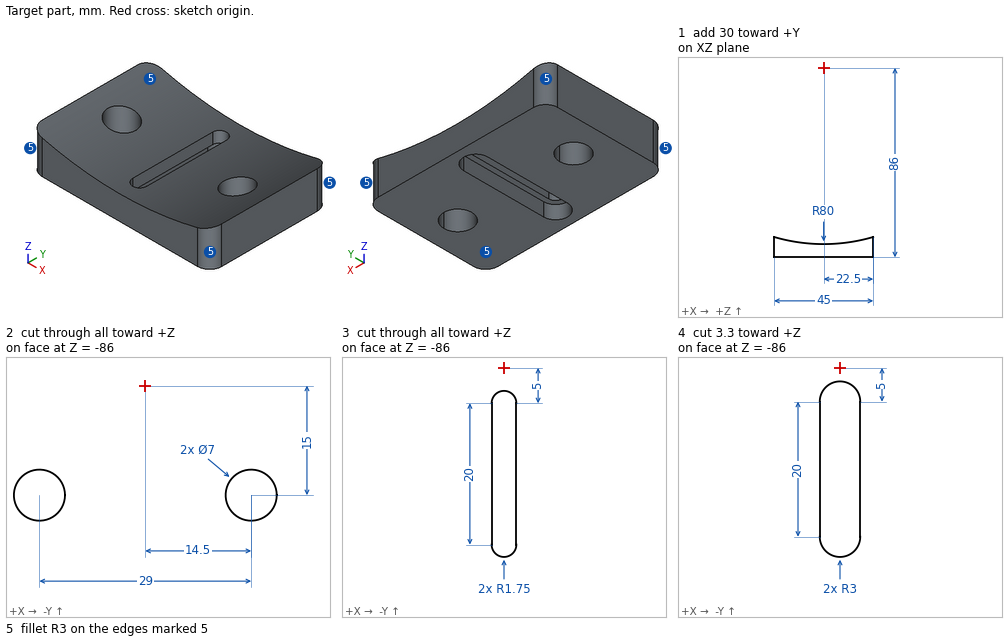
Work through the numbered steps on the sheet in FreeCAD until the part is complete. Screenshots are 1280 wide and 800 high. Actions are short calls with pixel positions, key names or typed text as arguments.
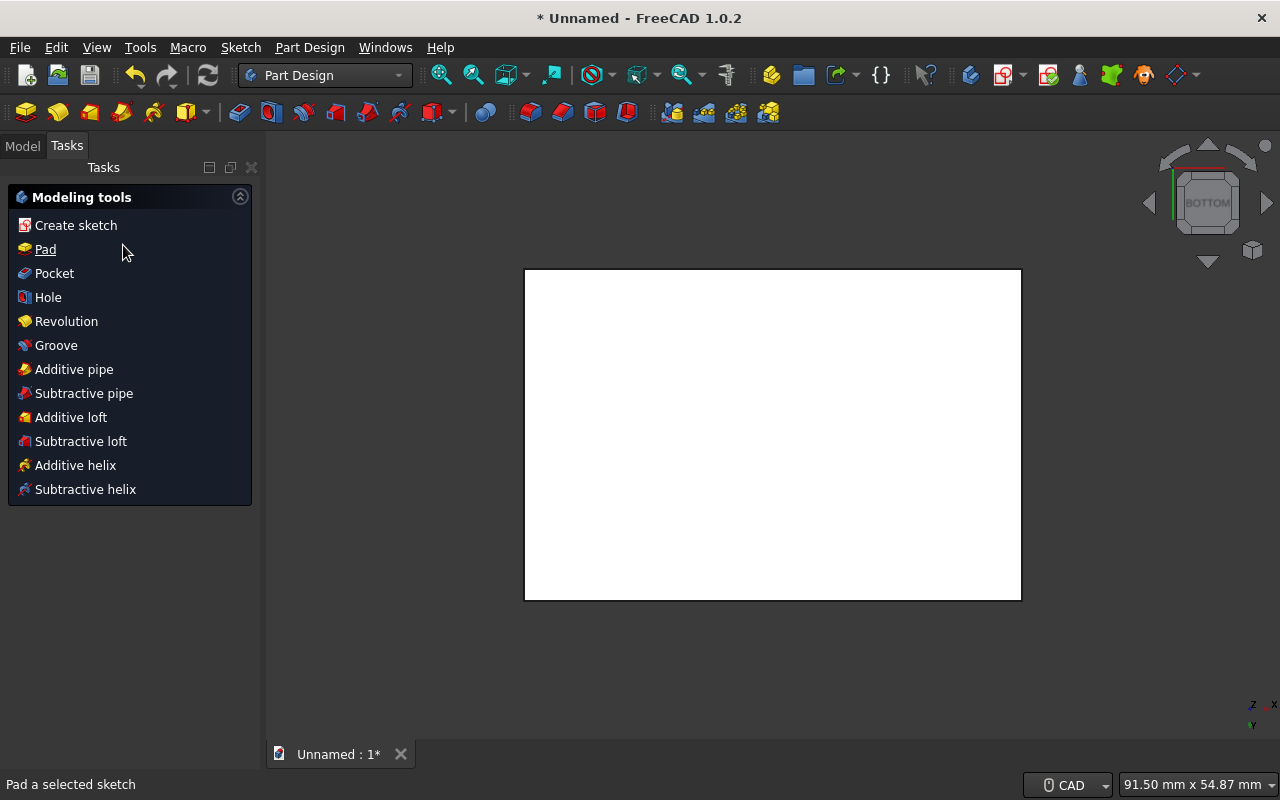
click(240, 112)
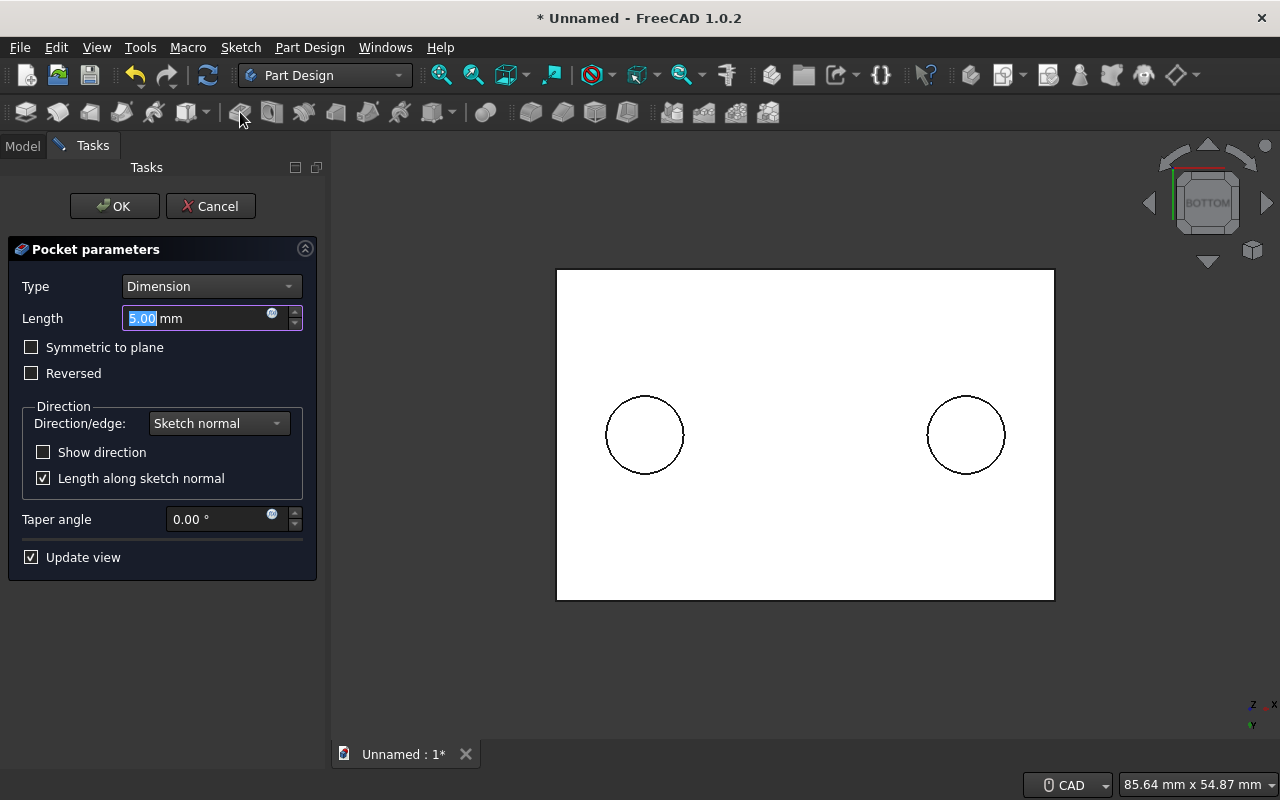
click(212, 286)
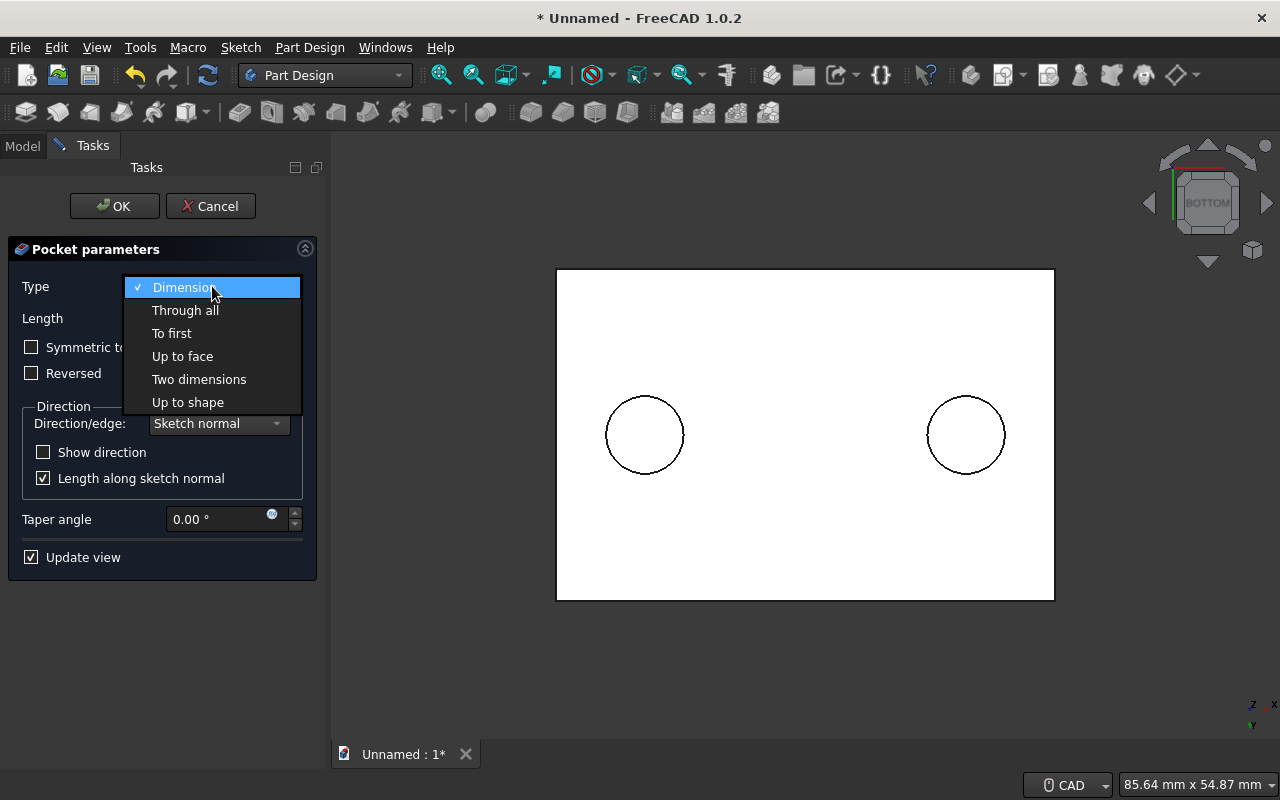
click(212, 310)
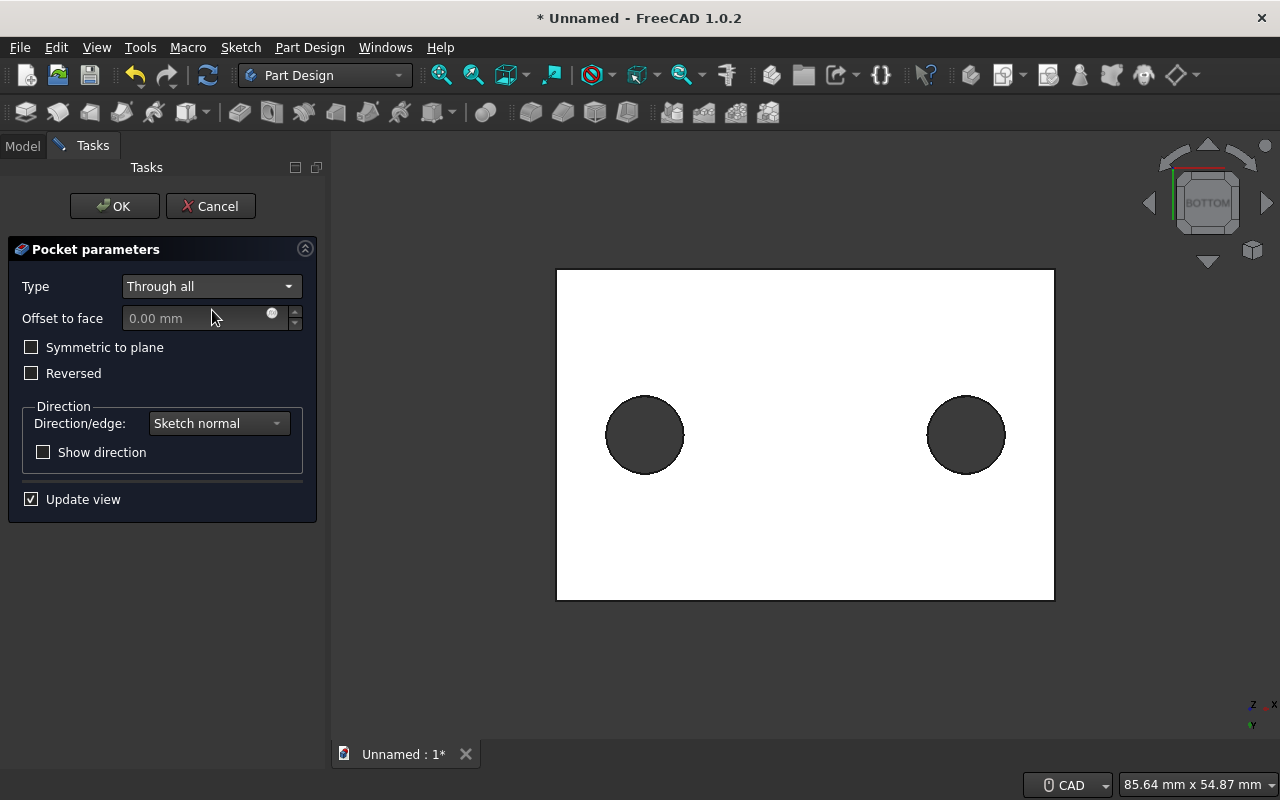
click(115, 206)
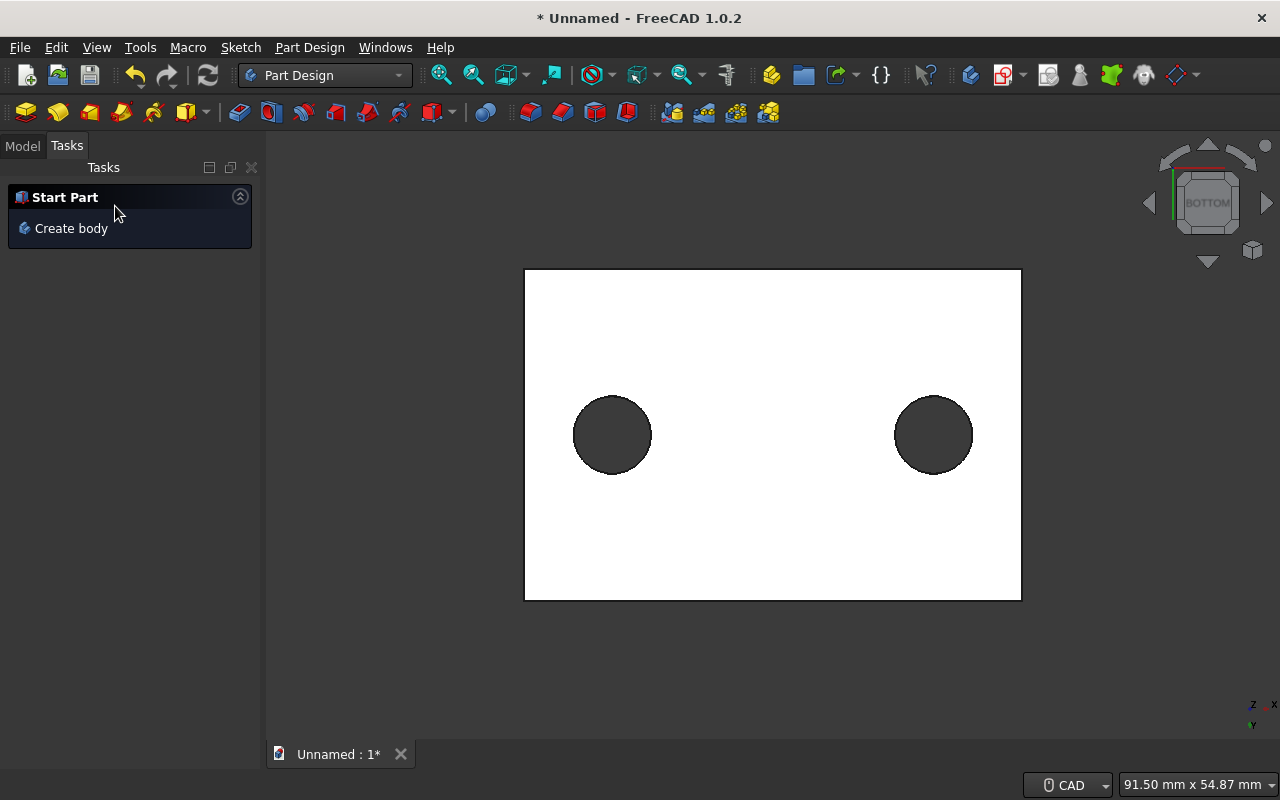
click(773, 434)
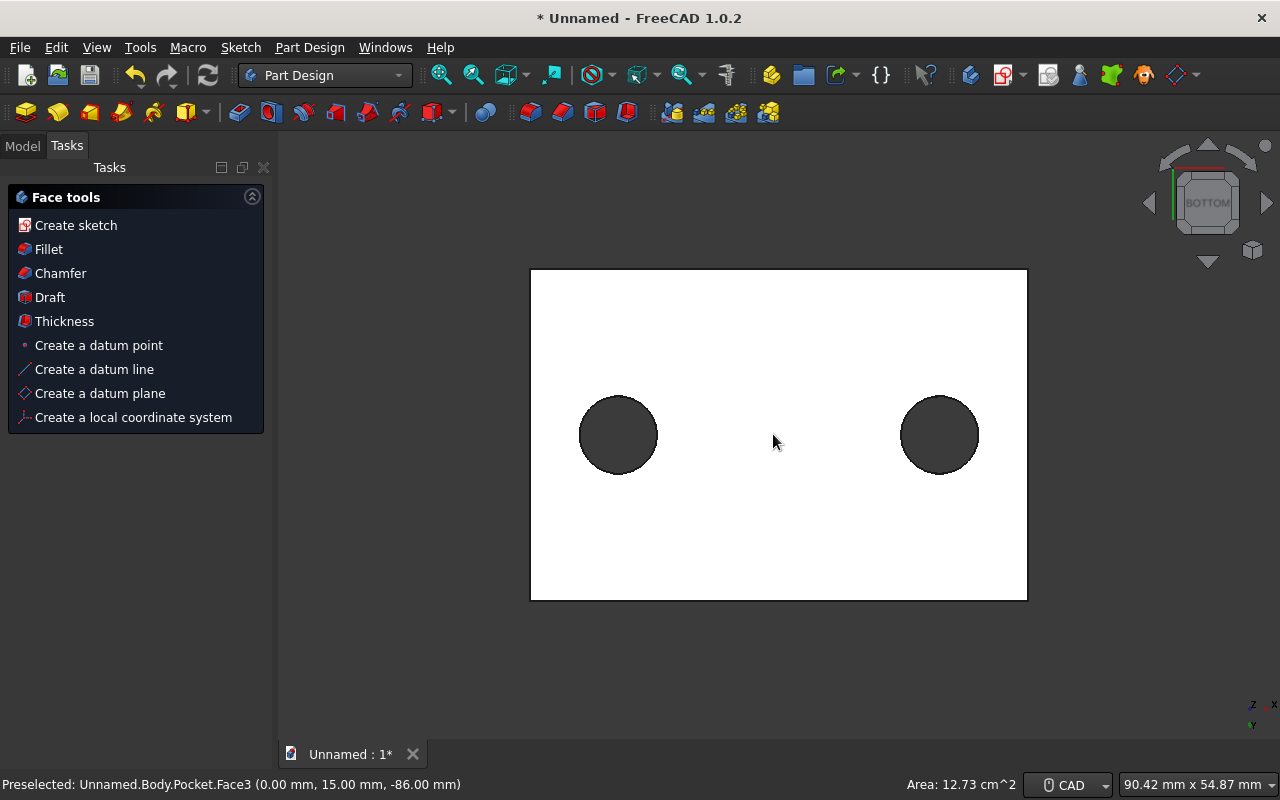
click(1004, 76)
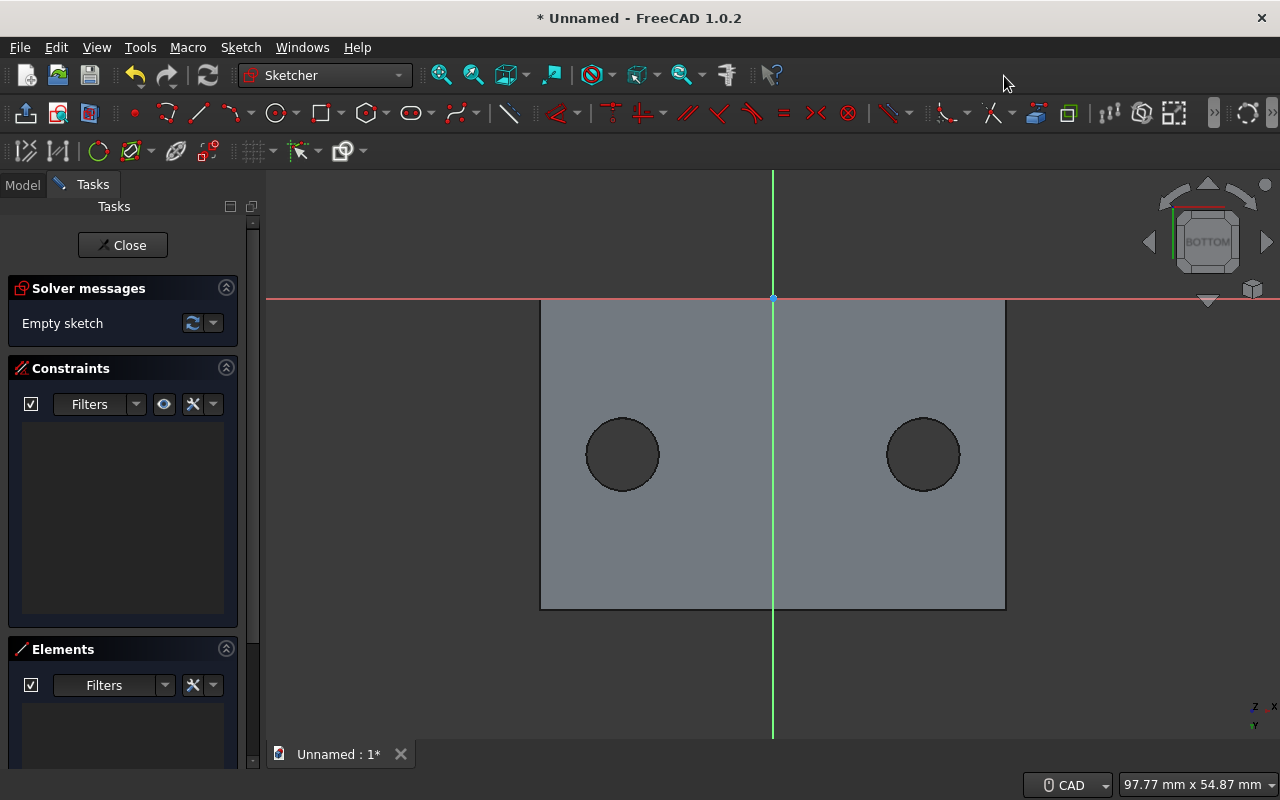
click(412, 114)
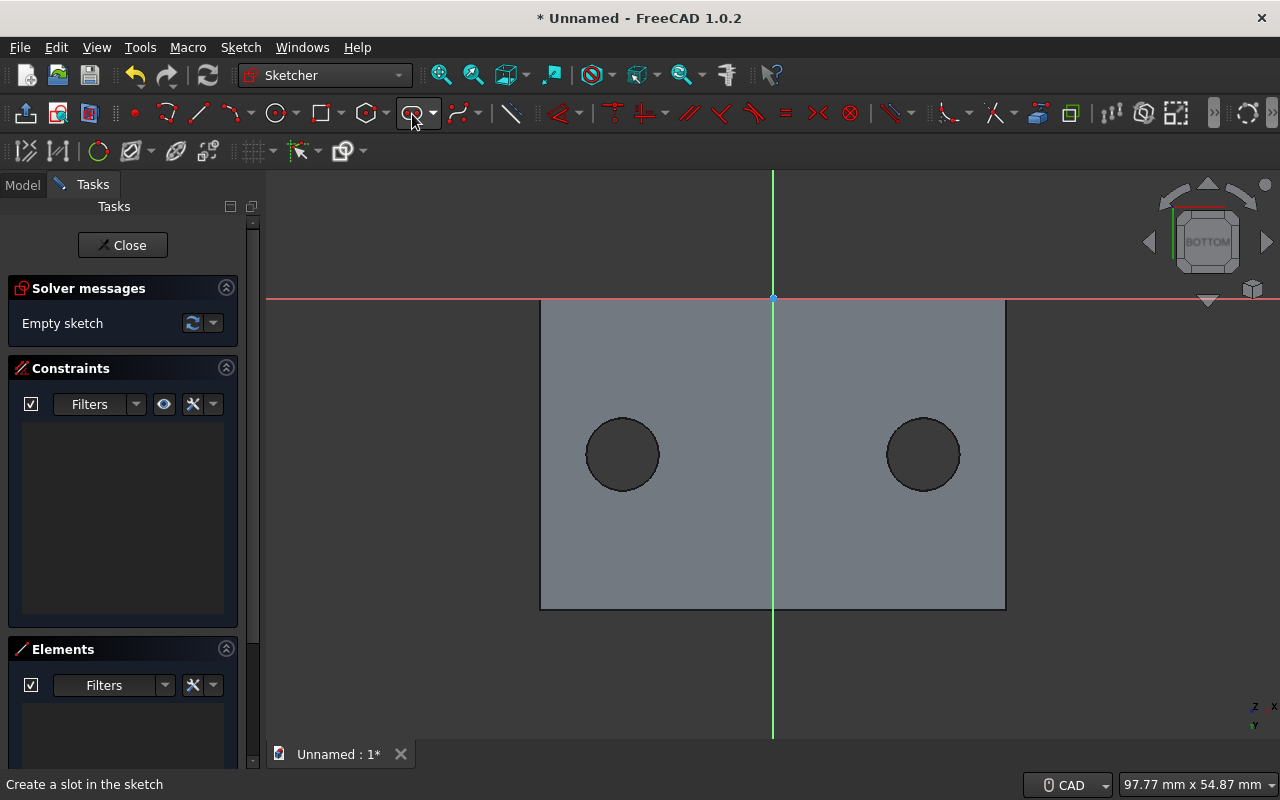
scroll(773, 558, up, 2)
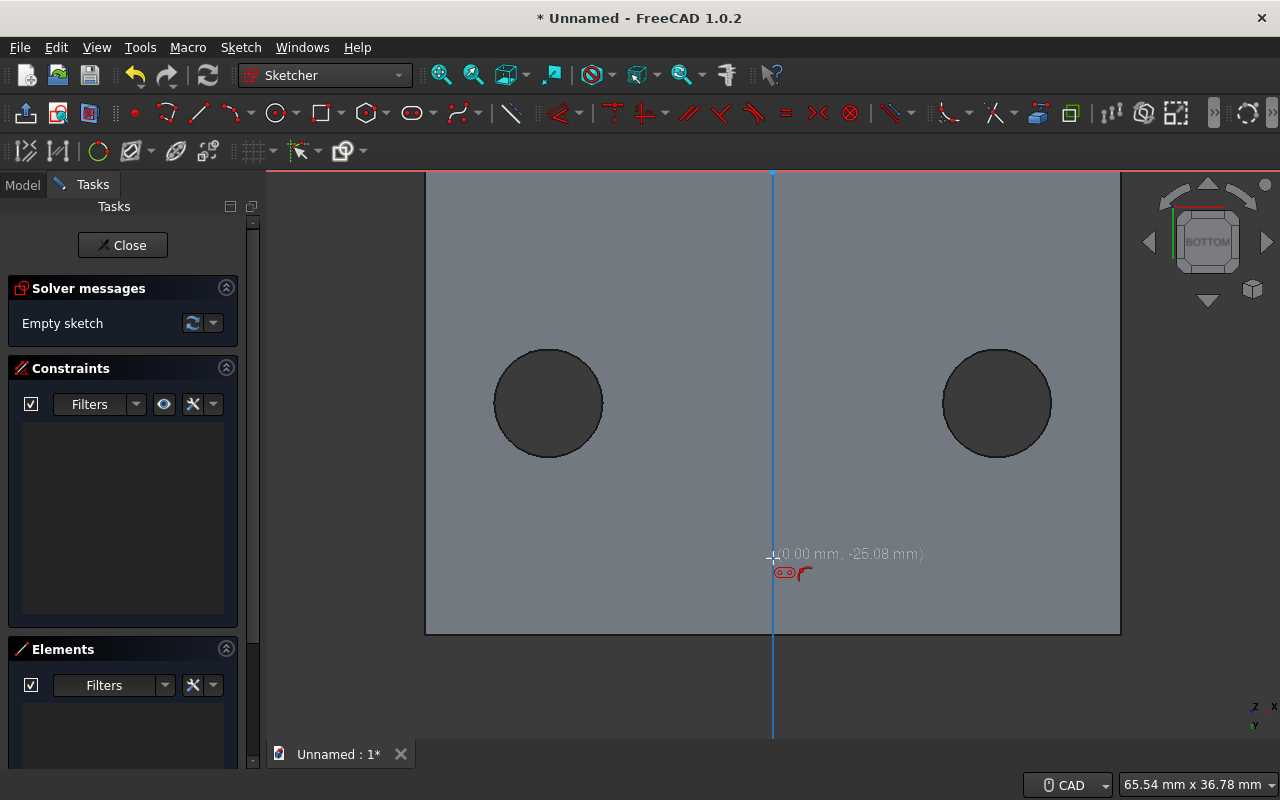
click(773, 558)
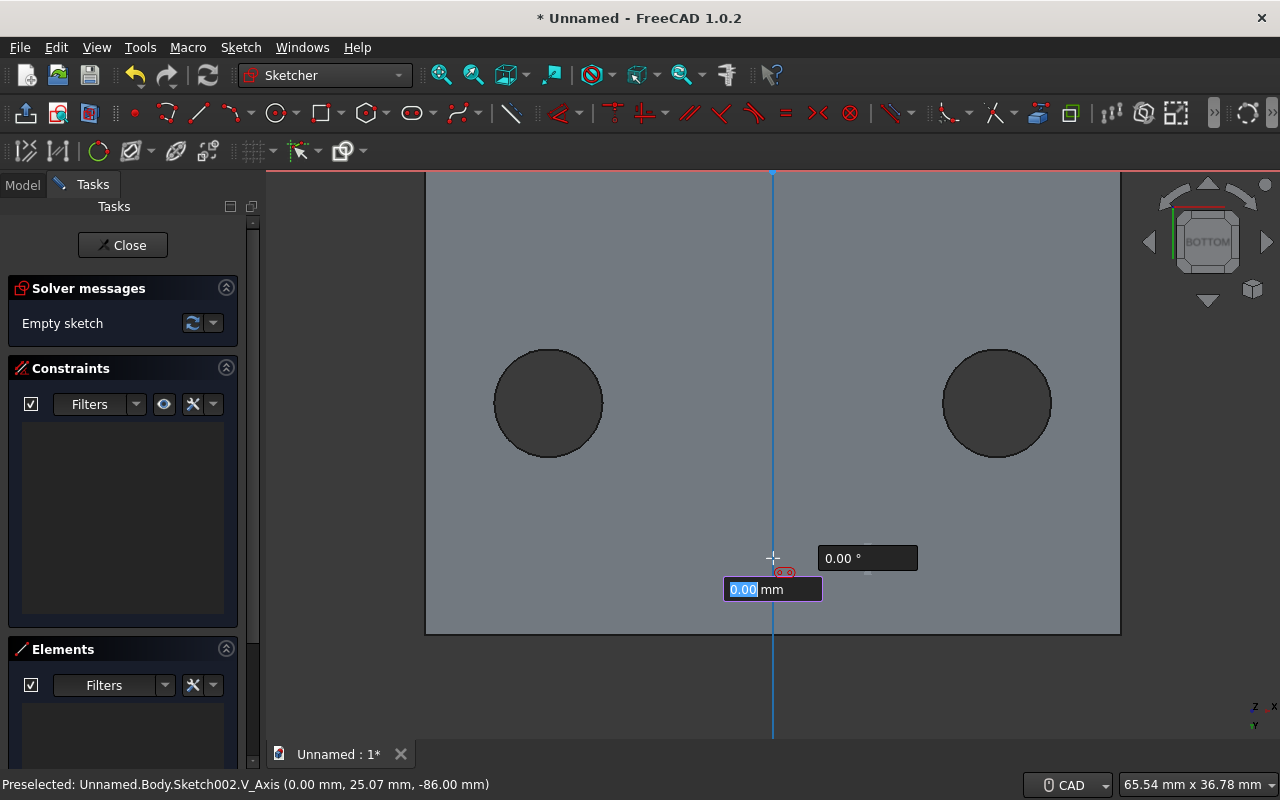
click(782, 249)